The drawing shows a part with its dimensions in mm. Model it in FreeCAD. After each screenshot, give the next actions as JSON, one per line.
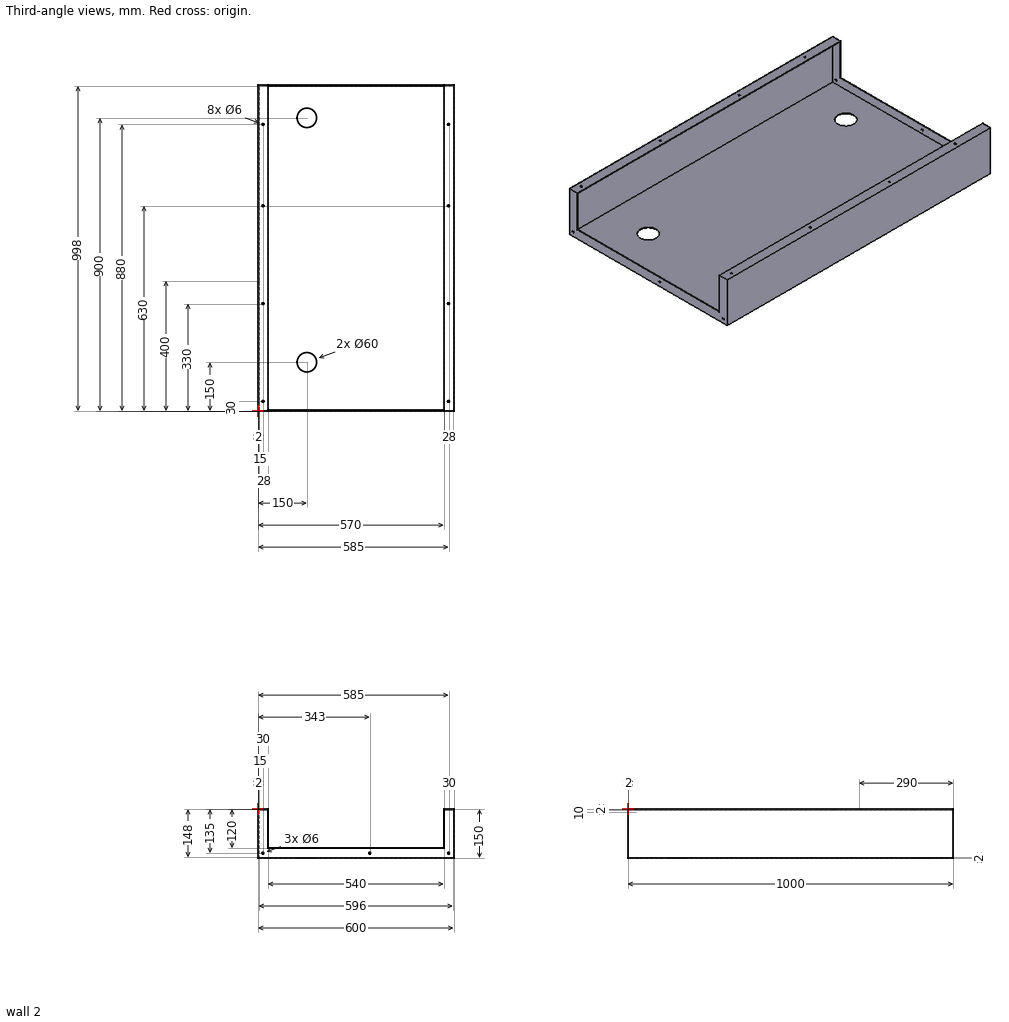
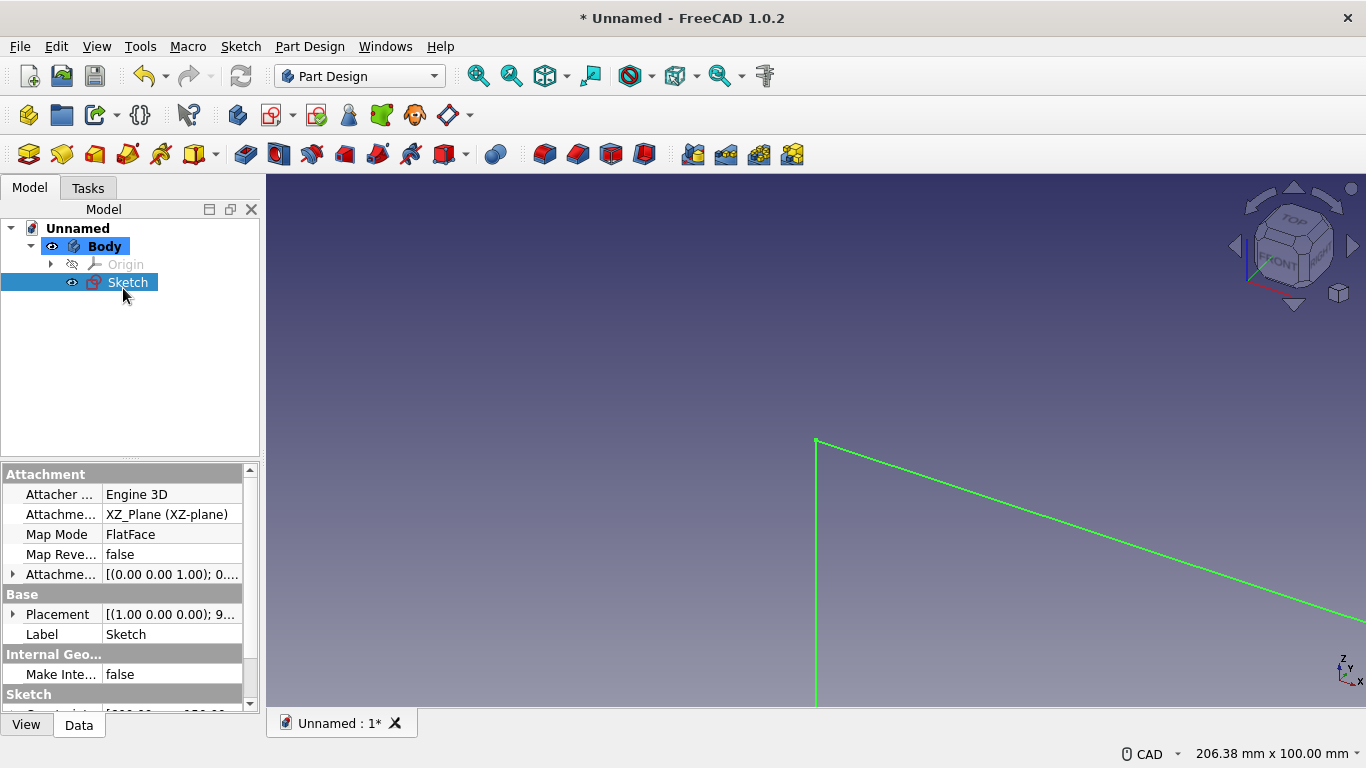
{"action": "left_click", "coordinate": [29, 154]}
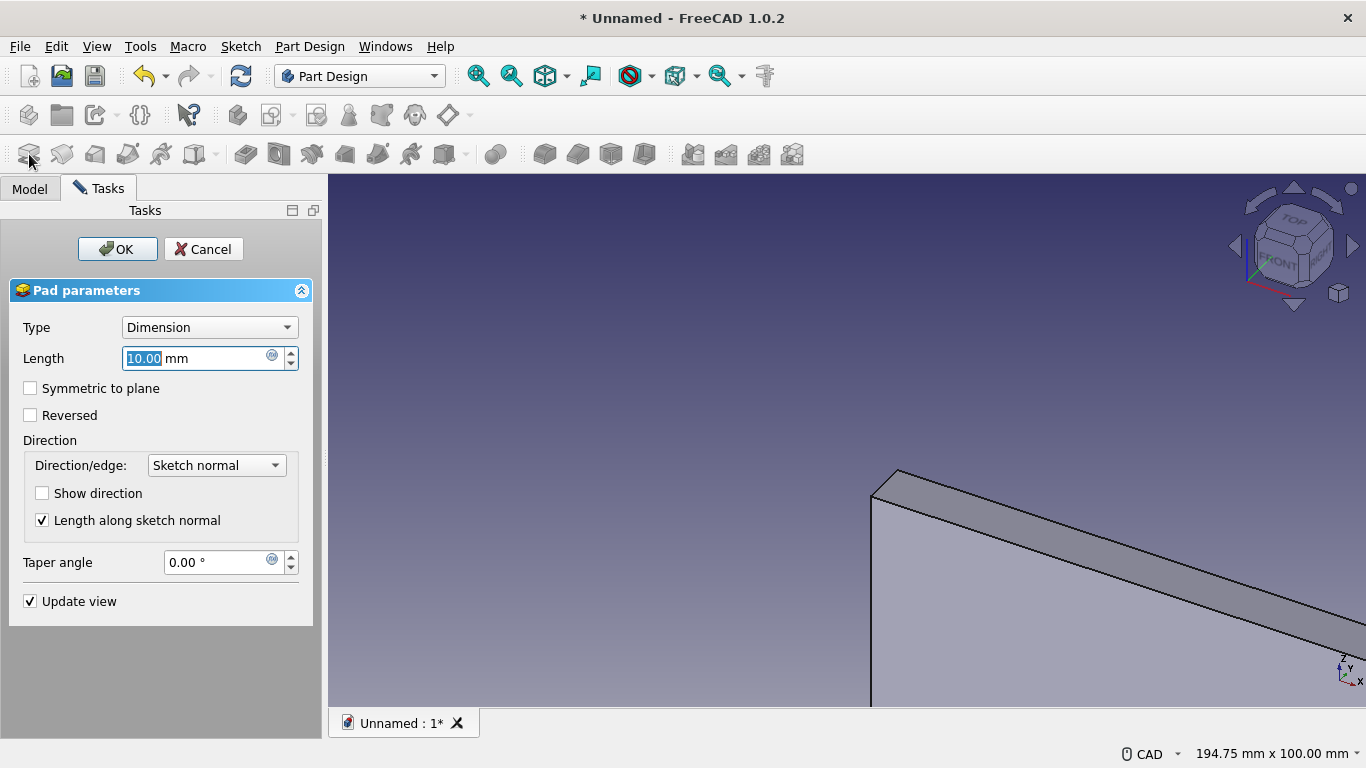
{"action": "type", "text": "1000"}
{"action": "key", "text": "Tab"}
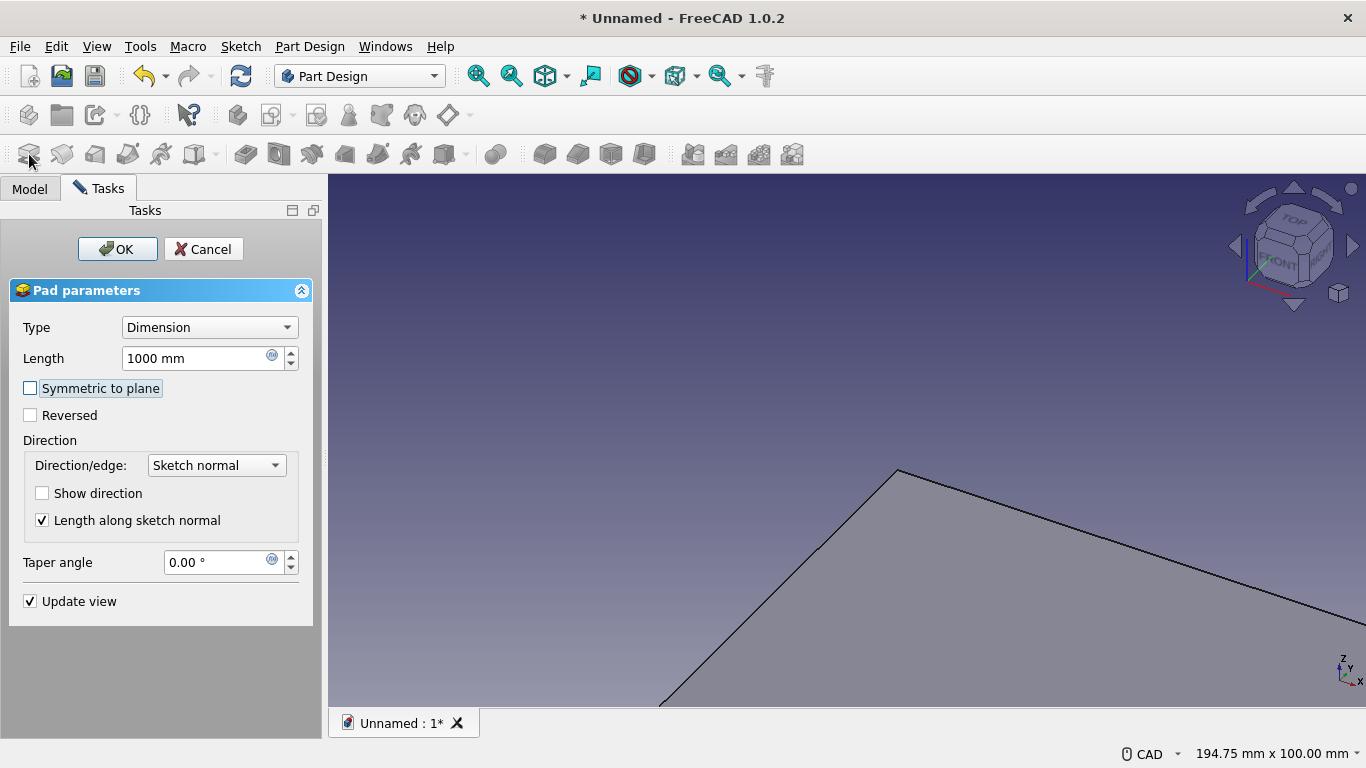
{"action": "left_click", "coordinate": [31, 415]}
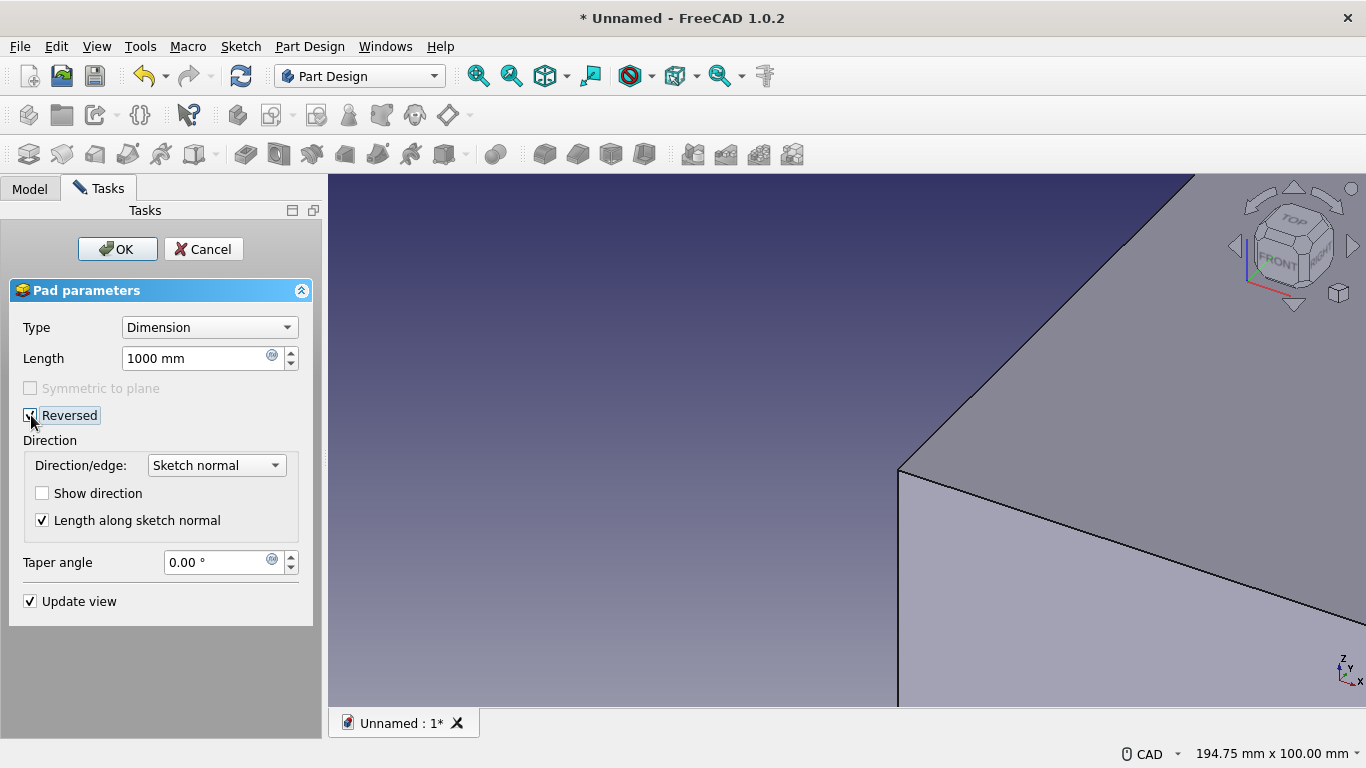
{"action": "left_click", "coordinate": [118, 249]}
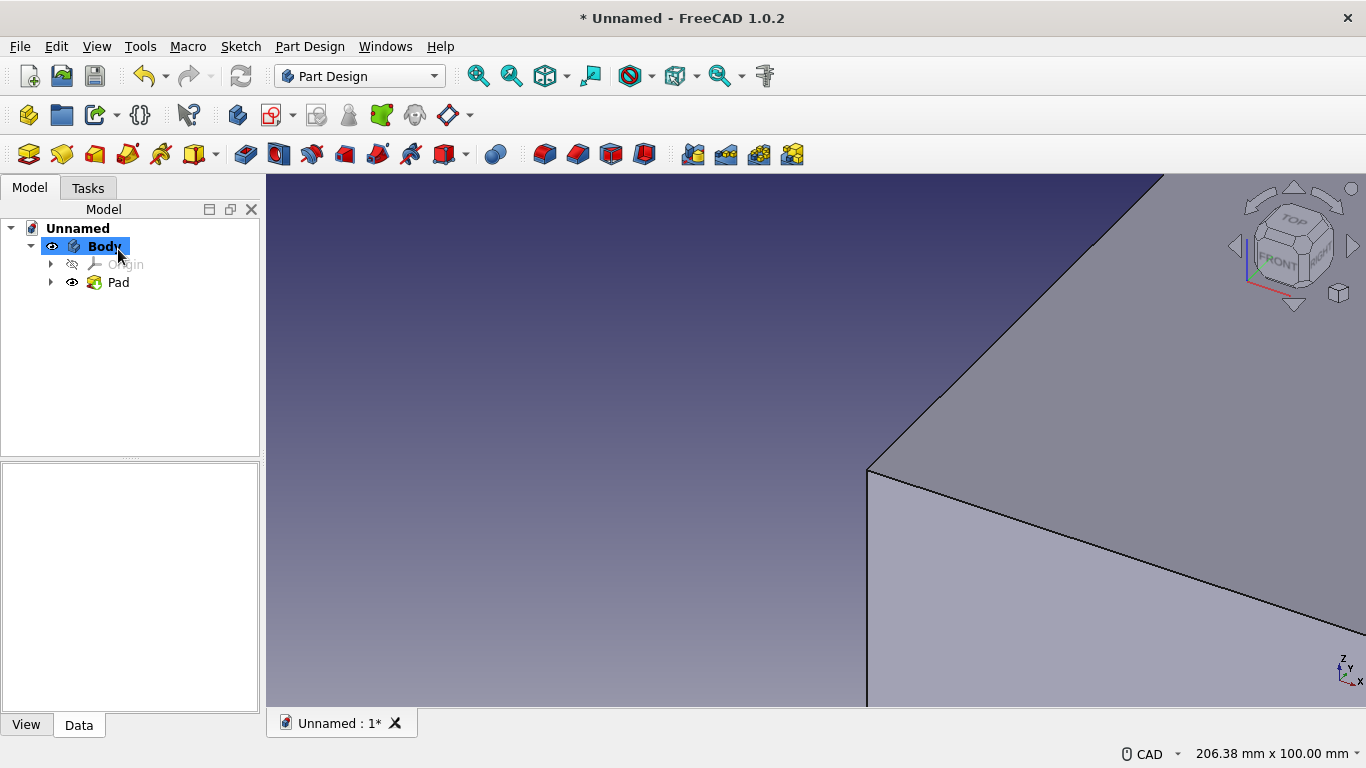
{"action": "left_click", "coordinate": [479, 76]}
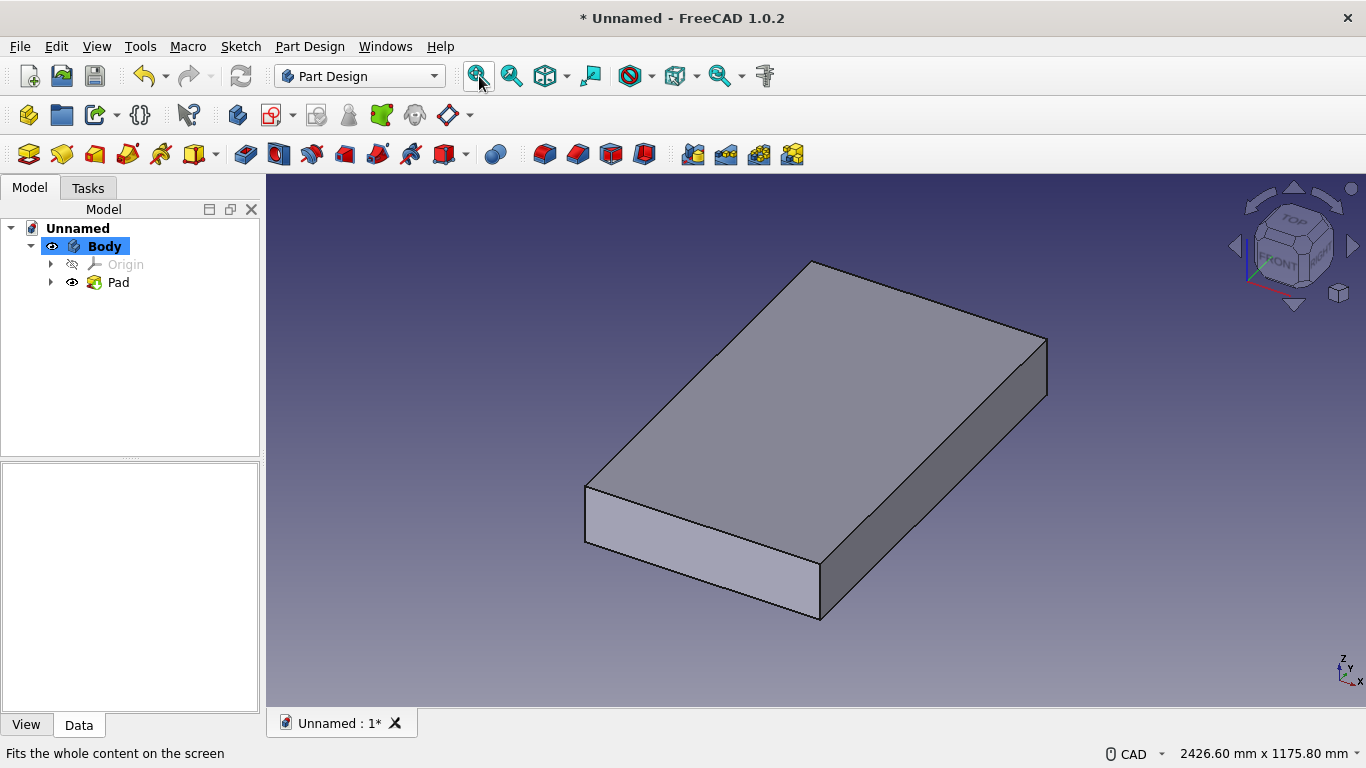
{"action": "left_click", "coordinate": [848, 379]}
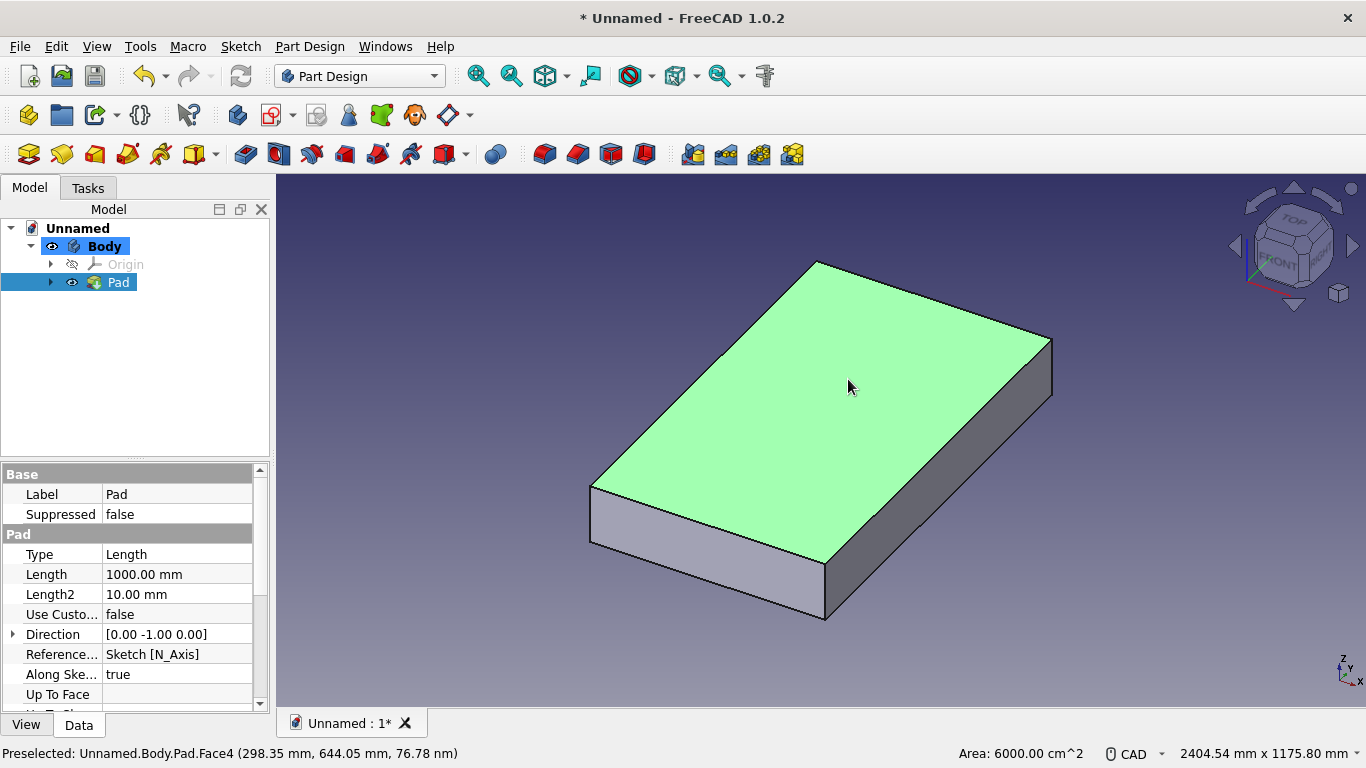
{"action": "left_click", "coordinate": [644, 154]}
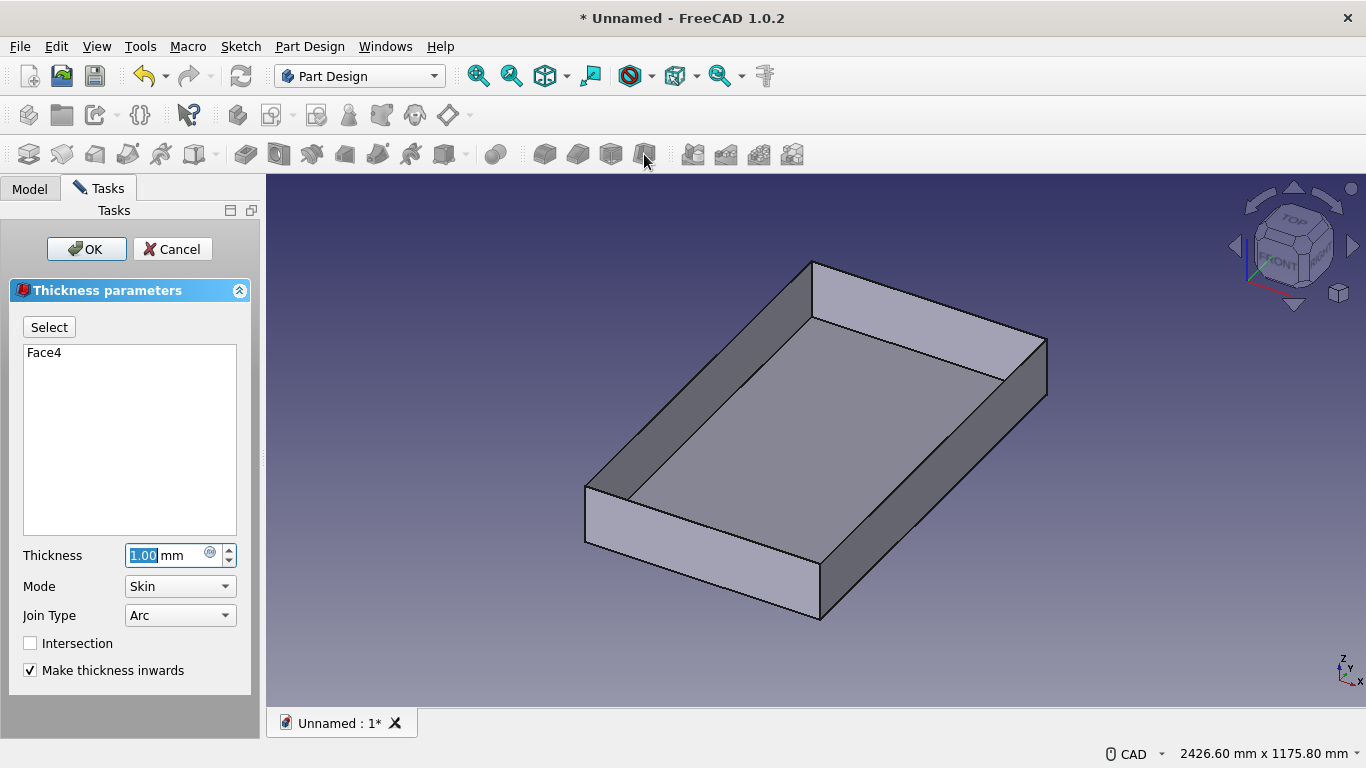
{"action": "type", "text": "2"}
{"action": "key", "text": "Tab"}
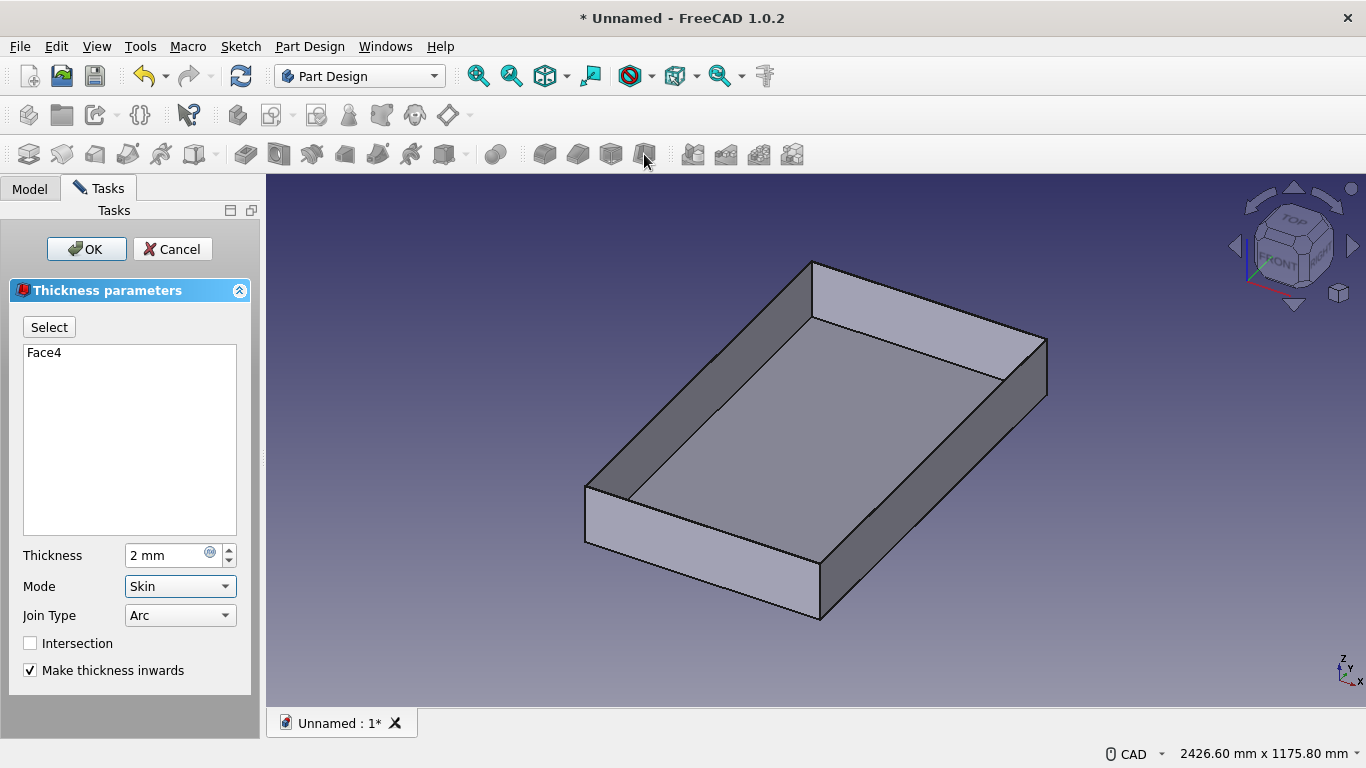
{"action": "left_click", "coordinate": [181, 616]}